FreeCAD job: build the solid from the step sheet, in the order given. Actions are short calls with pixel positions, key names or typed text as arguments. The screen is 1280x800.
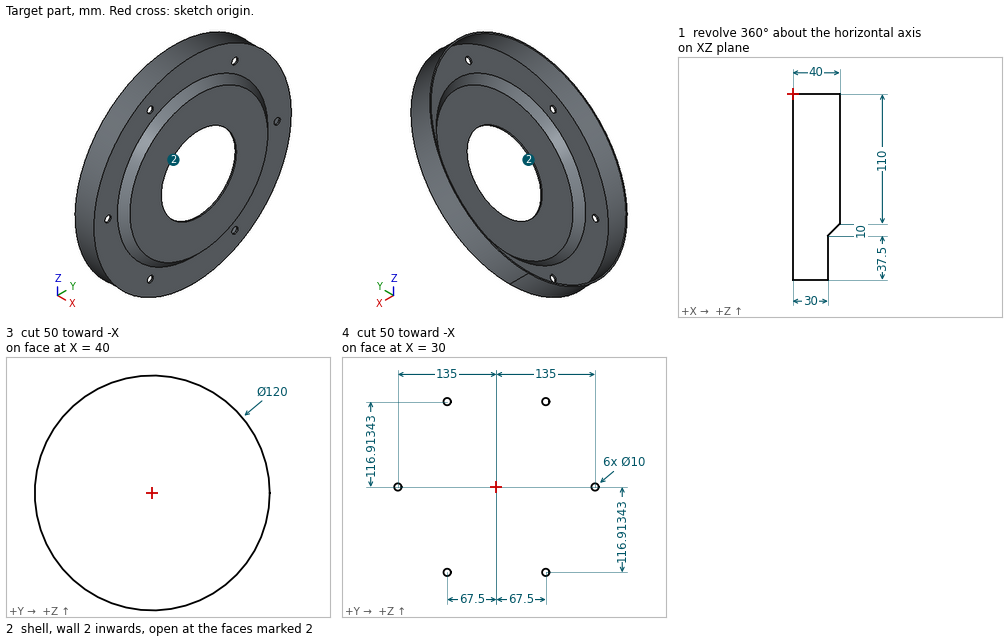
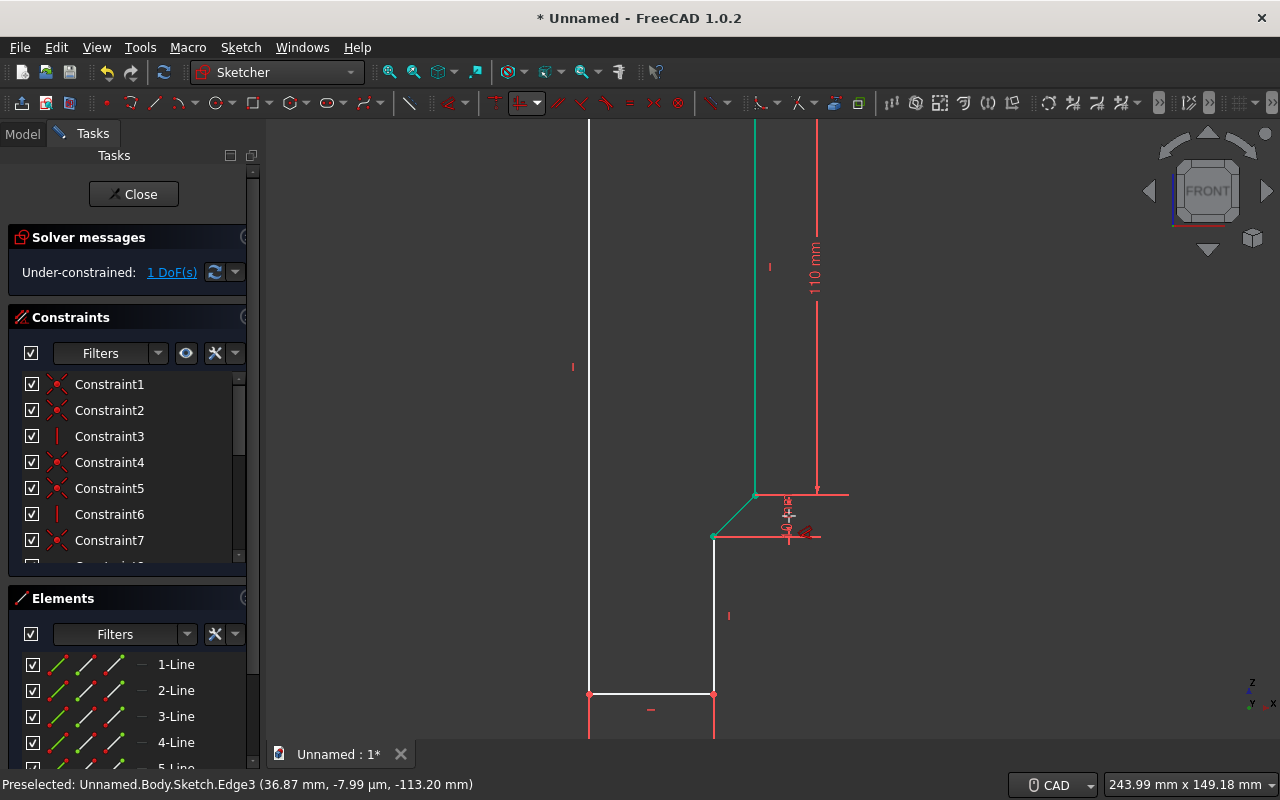
click(714, 584)
click(748, 616)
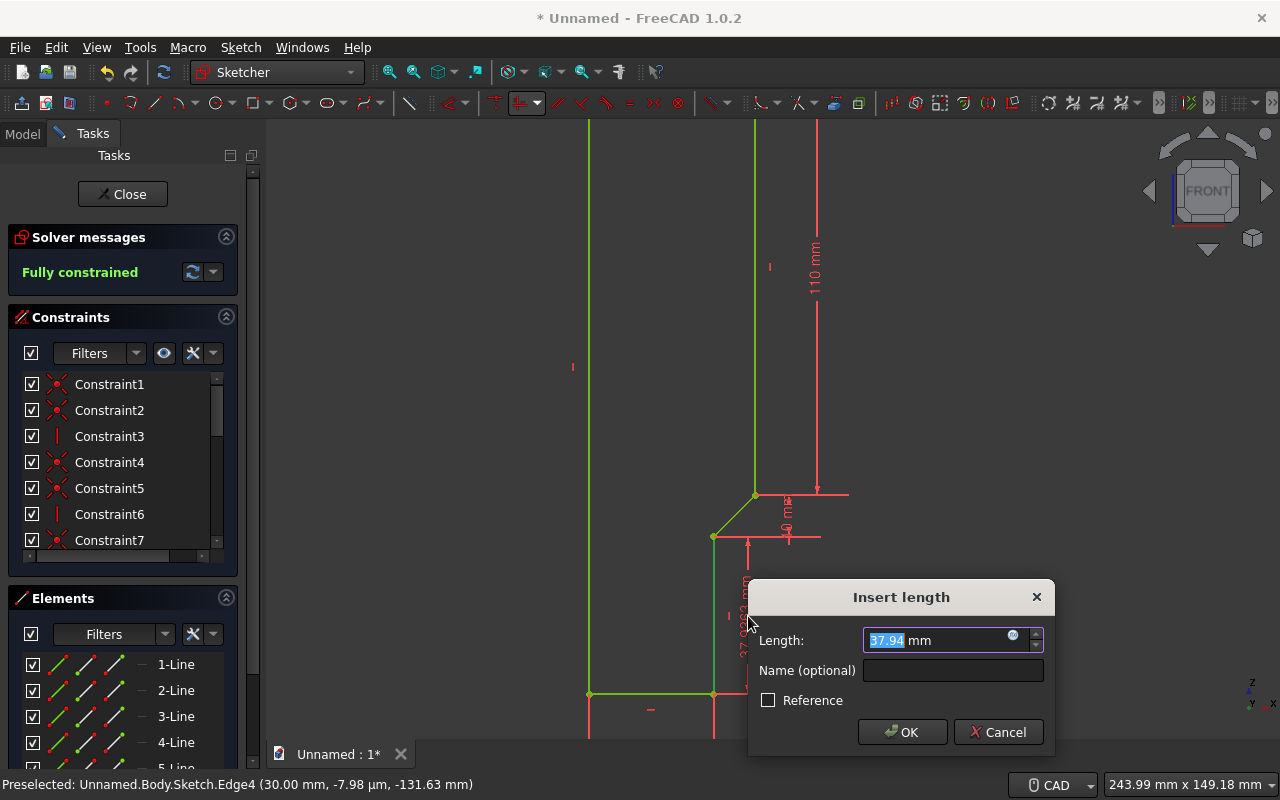
text(37.5)
key(Return)
key(Escape)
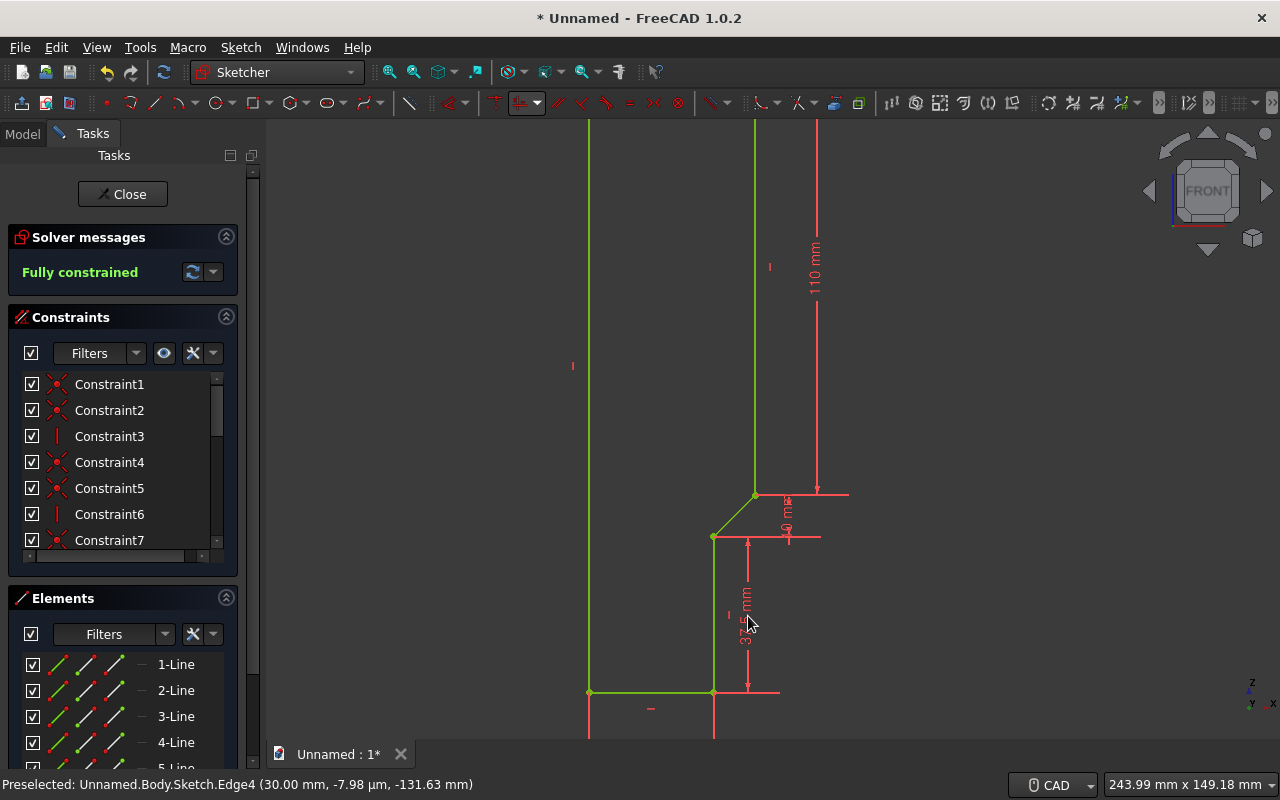
click(123, 194)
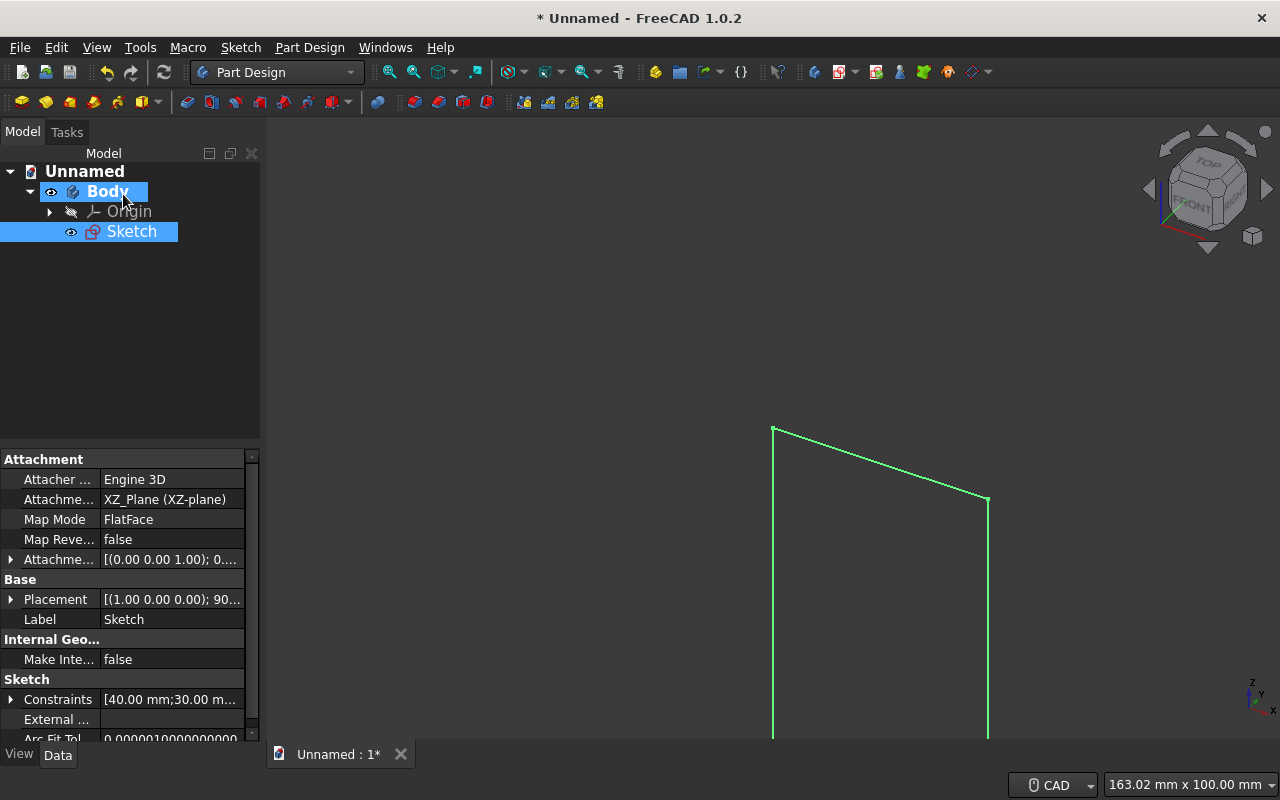
click(46, 102)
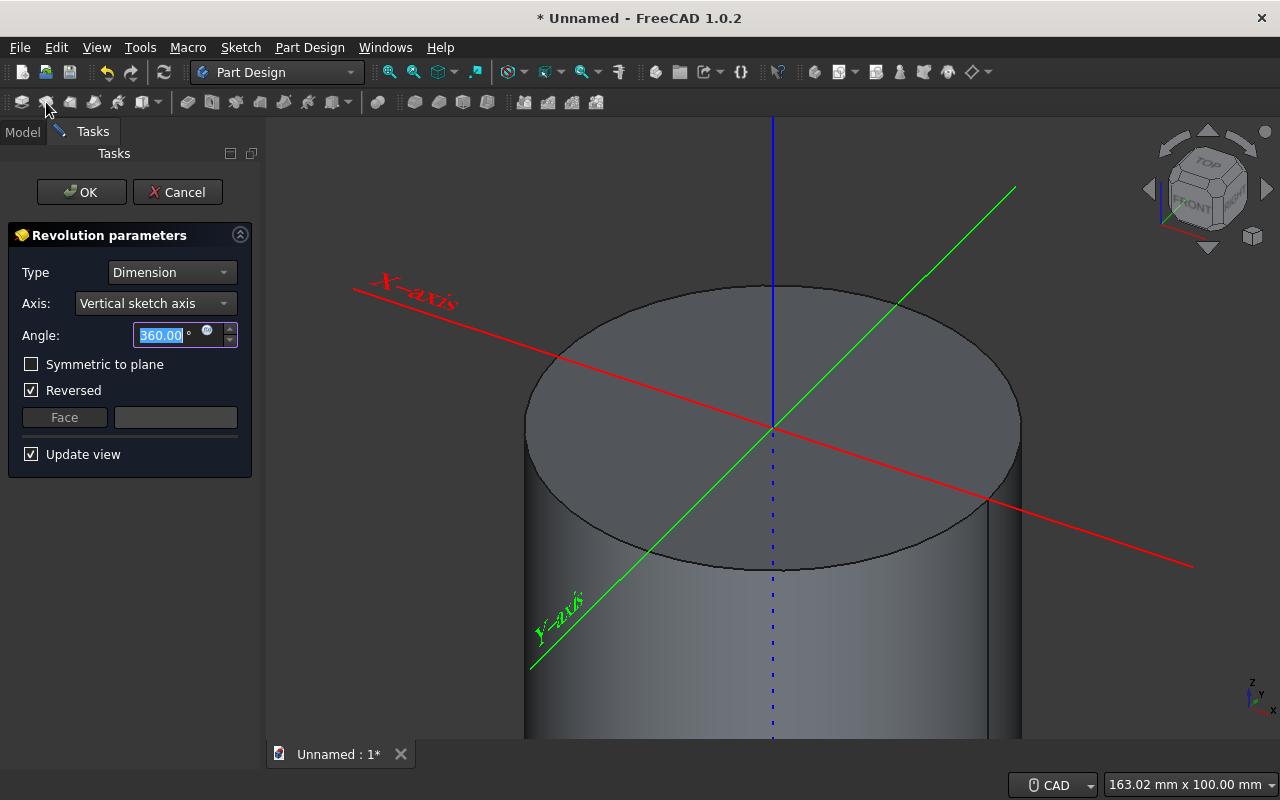
click(156, 304)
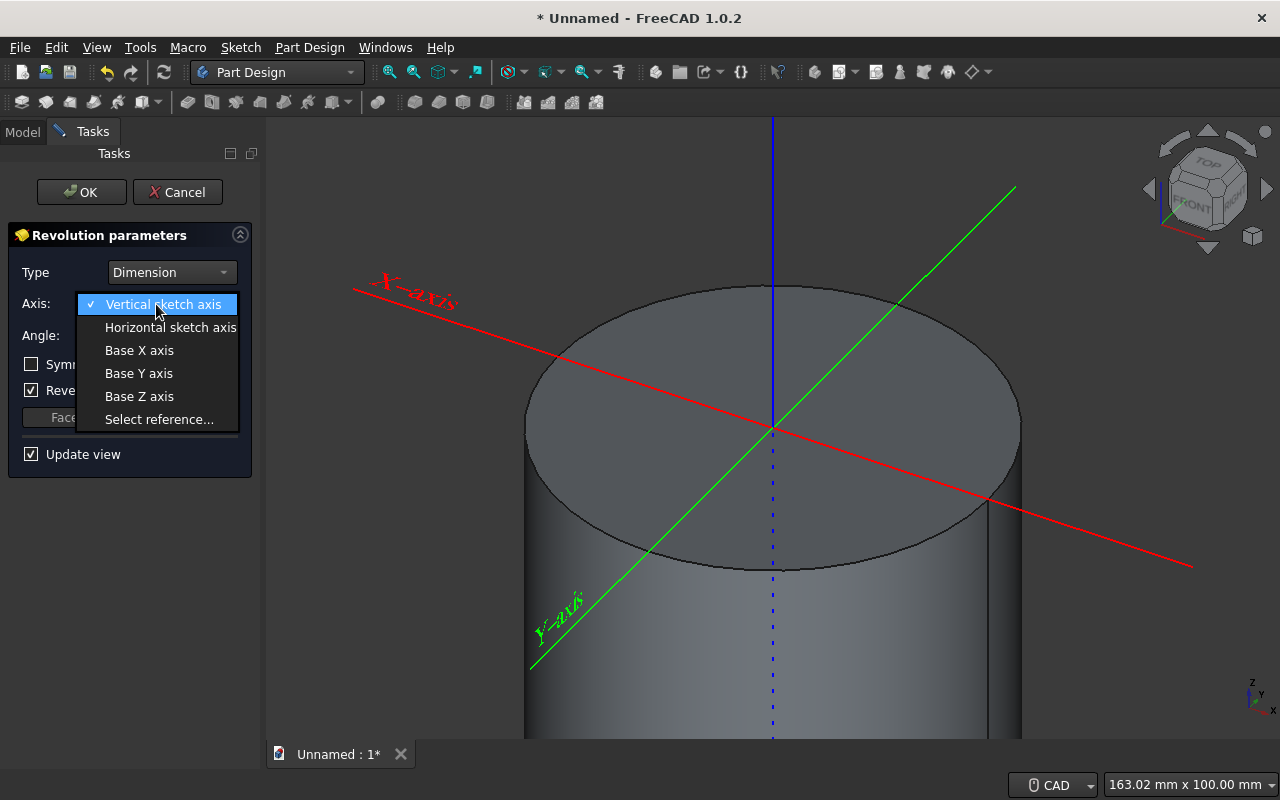
click(156, 328)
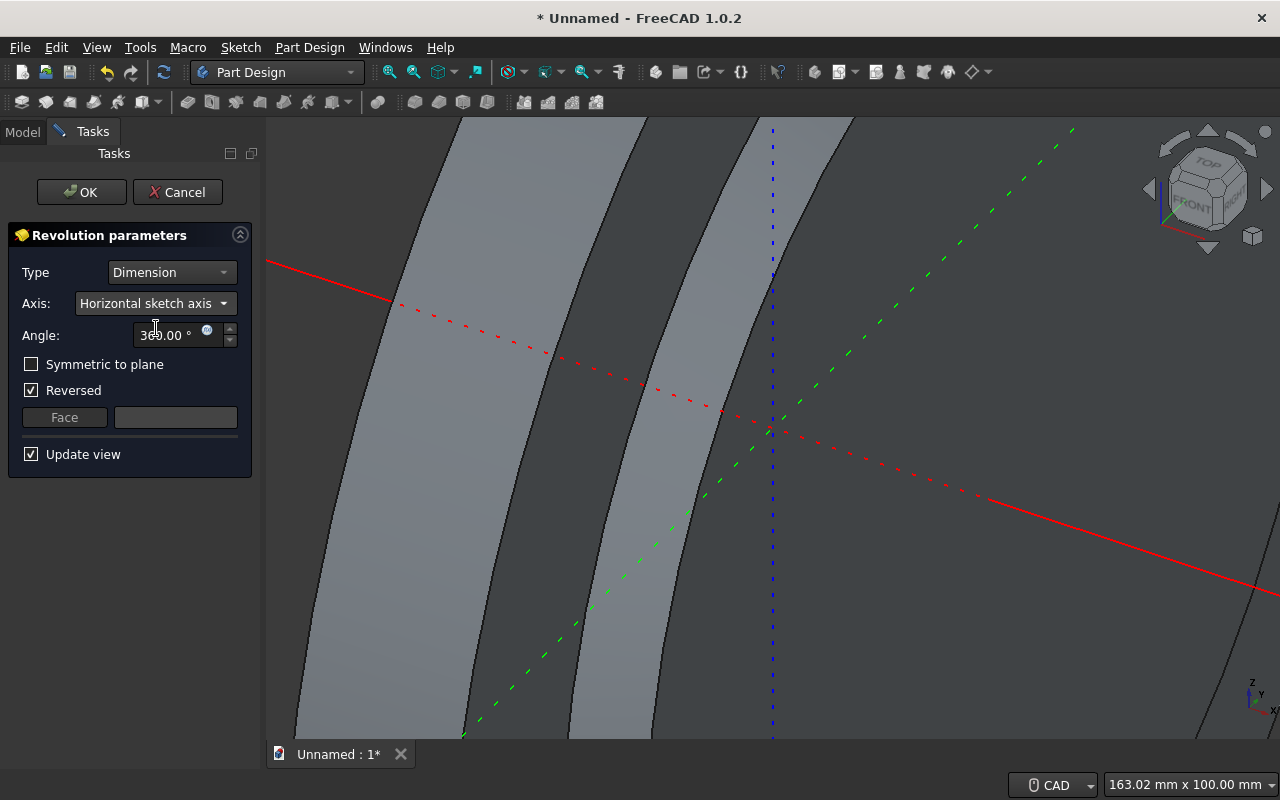
click(82, 192)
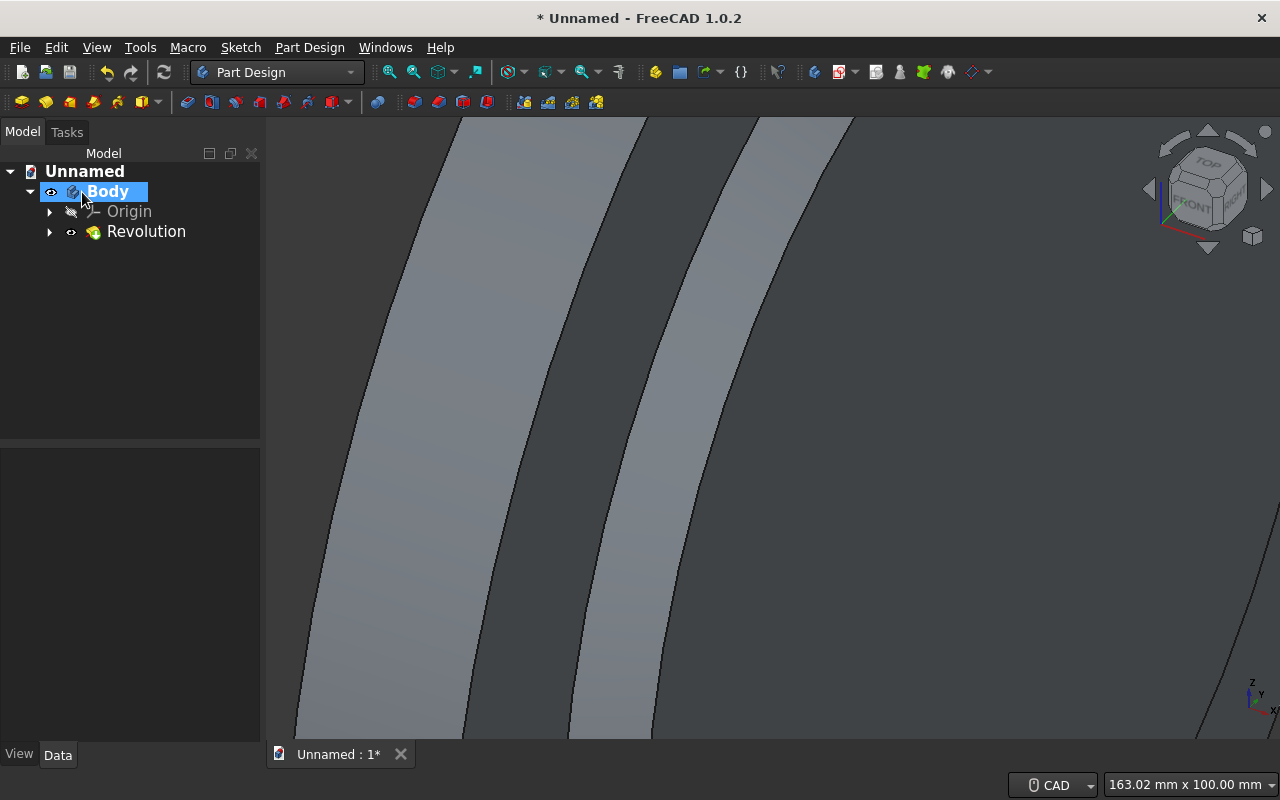
click(390, 72)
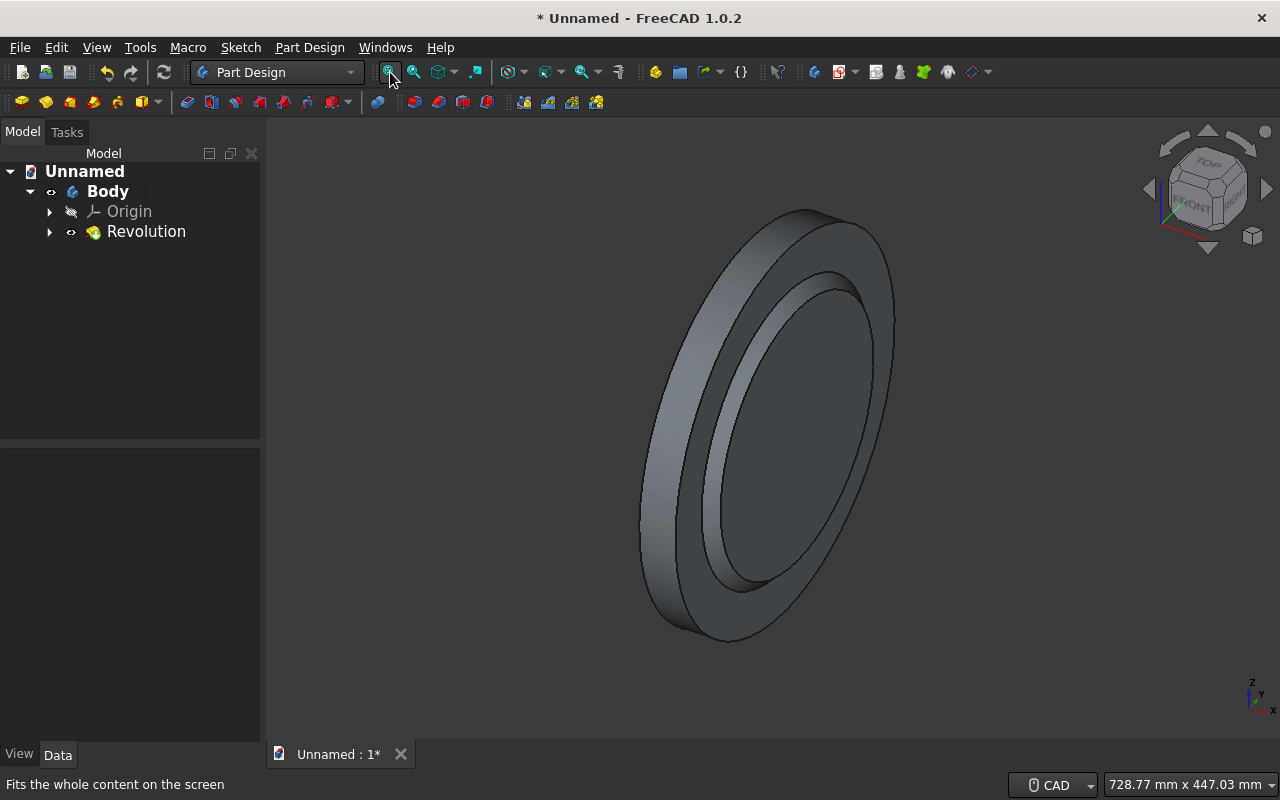
key(0)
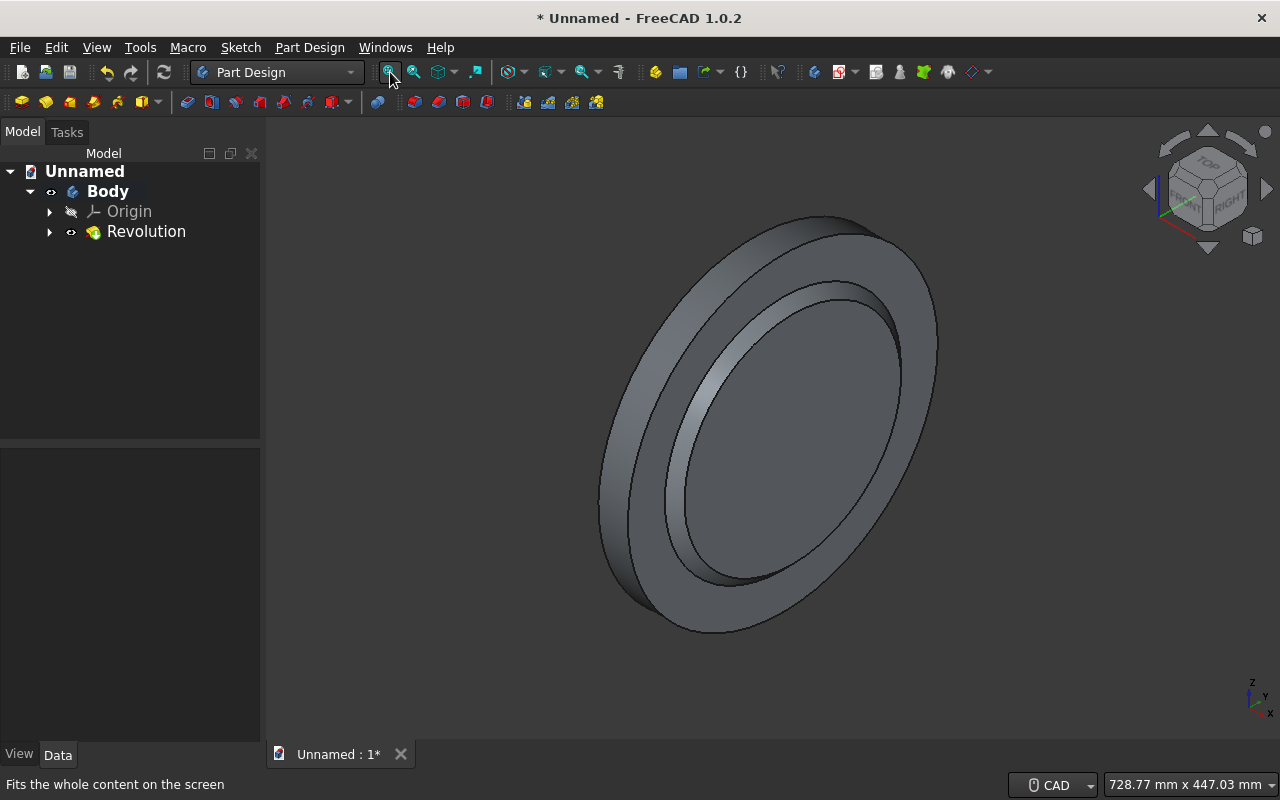
key(2)